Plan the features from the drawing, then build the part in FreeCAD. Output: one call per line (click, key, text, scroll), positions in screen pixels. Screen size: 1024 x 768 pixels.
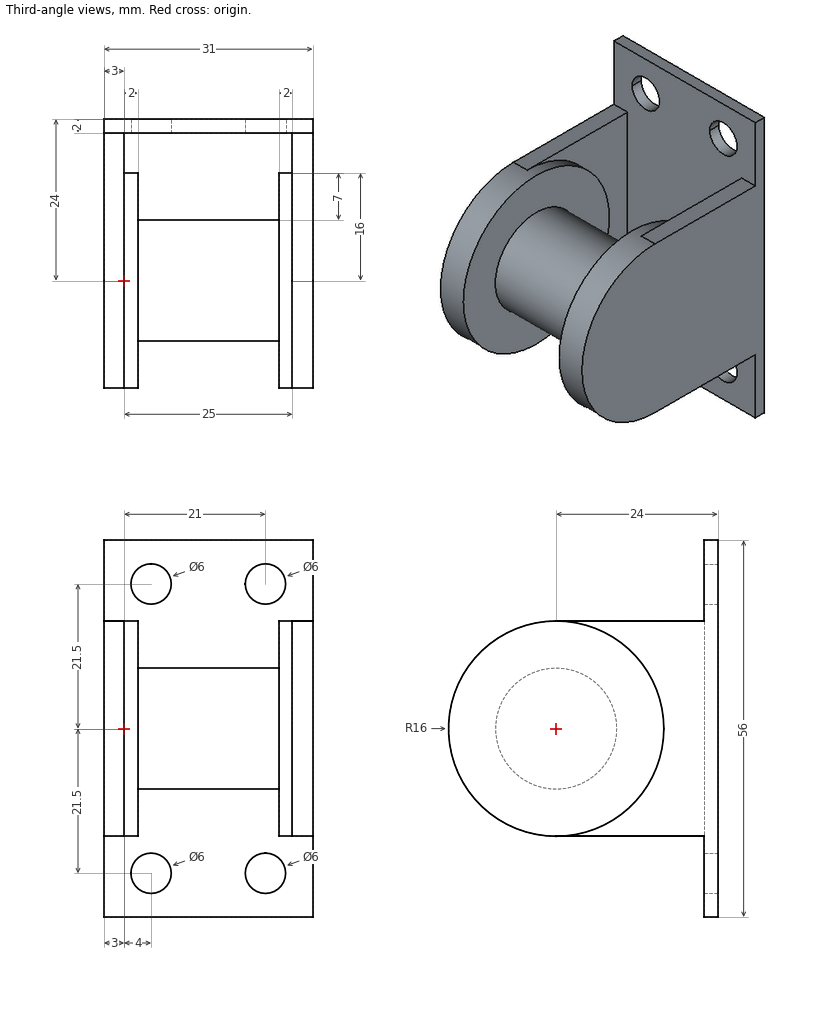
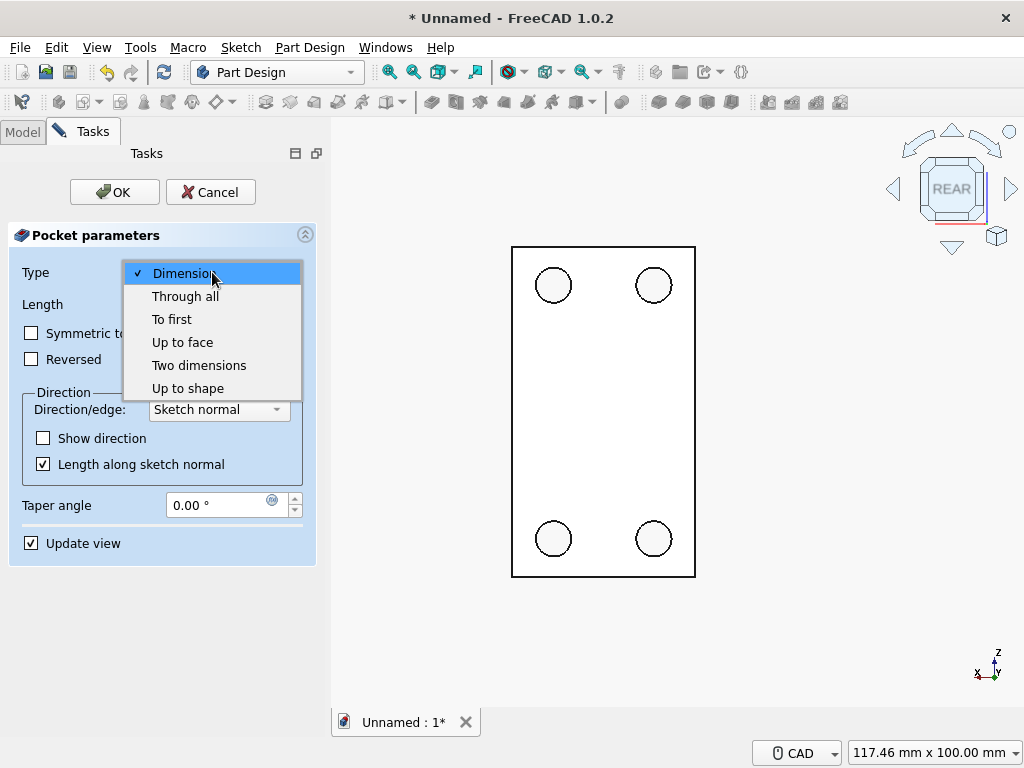
click(212, 320)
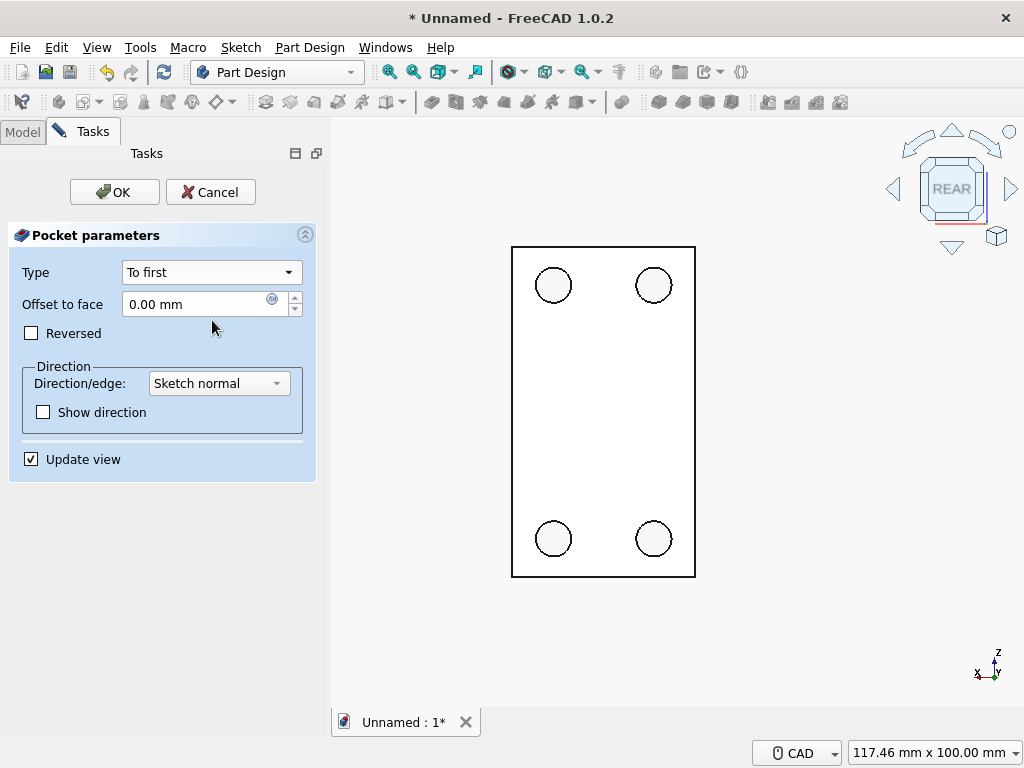
click(115, 192)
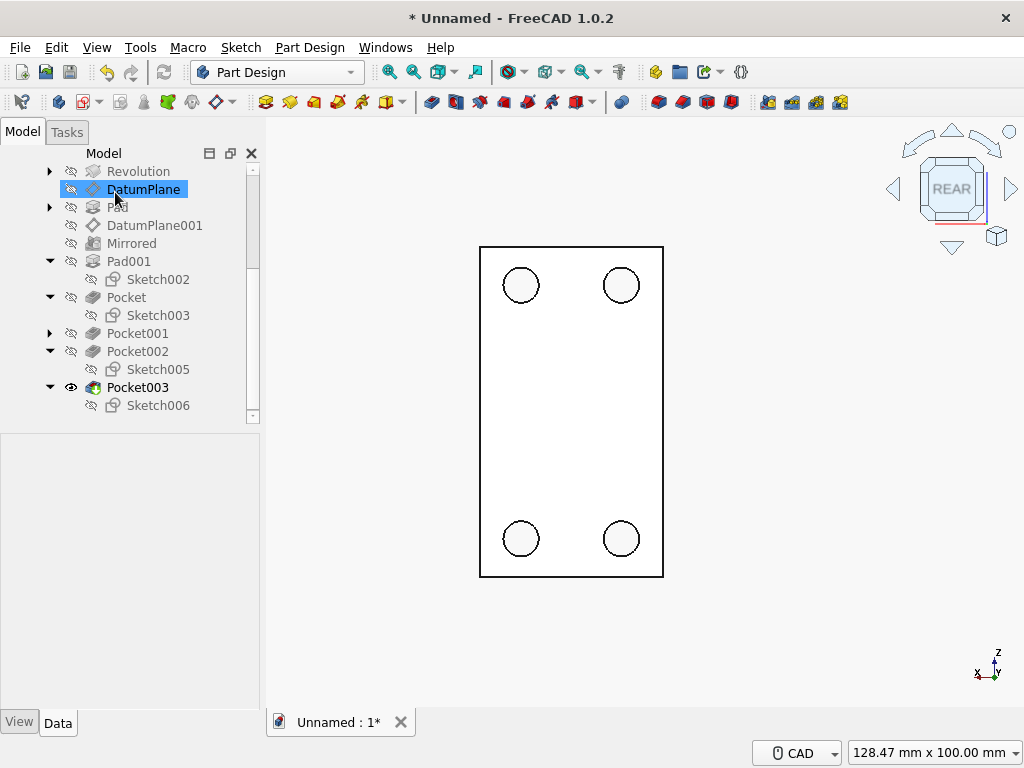
key(0)